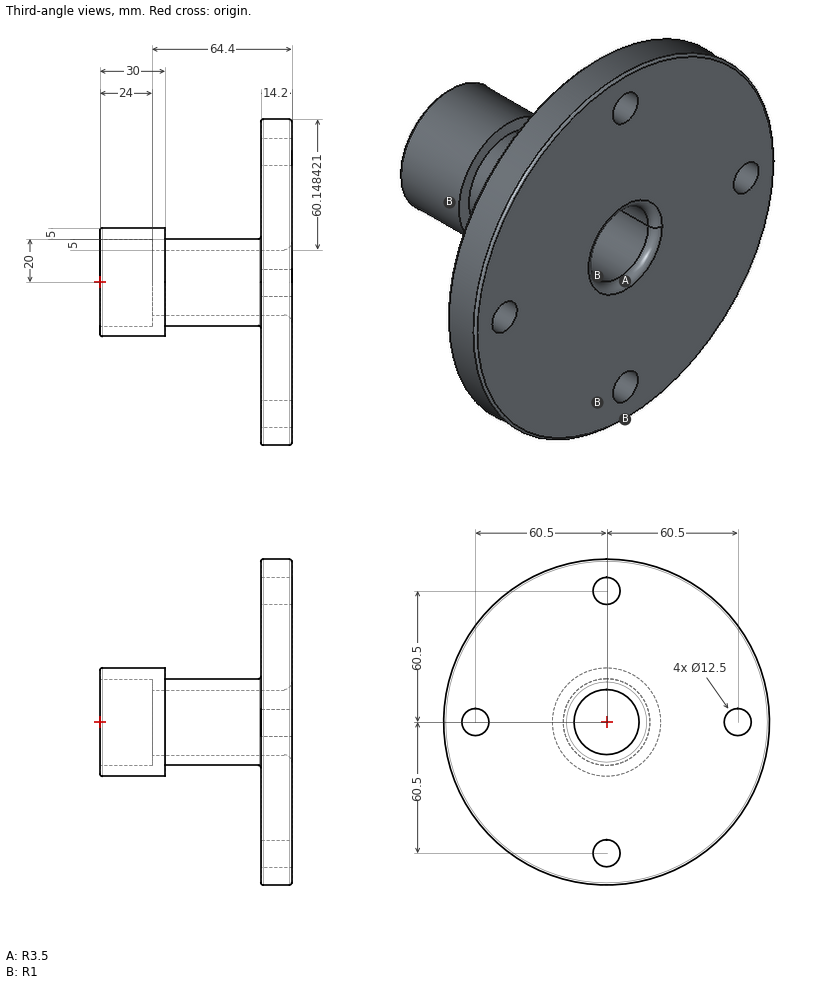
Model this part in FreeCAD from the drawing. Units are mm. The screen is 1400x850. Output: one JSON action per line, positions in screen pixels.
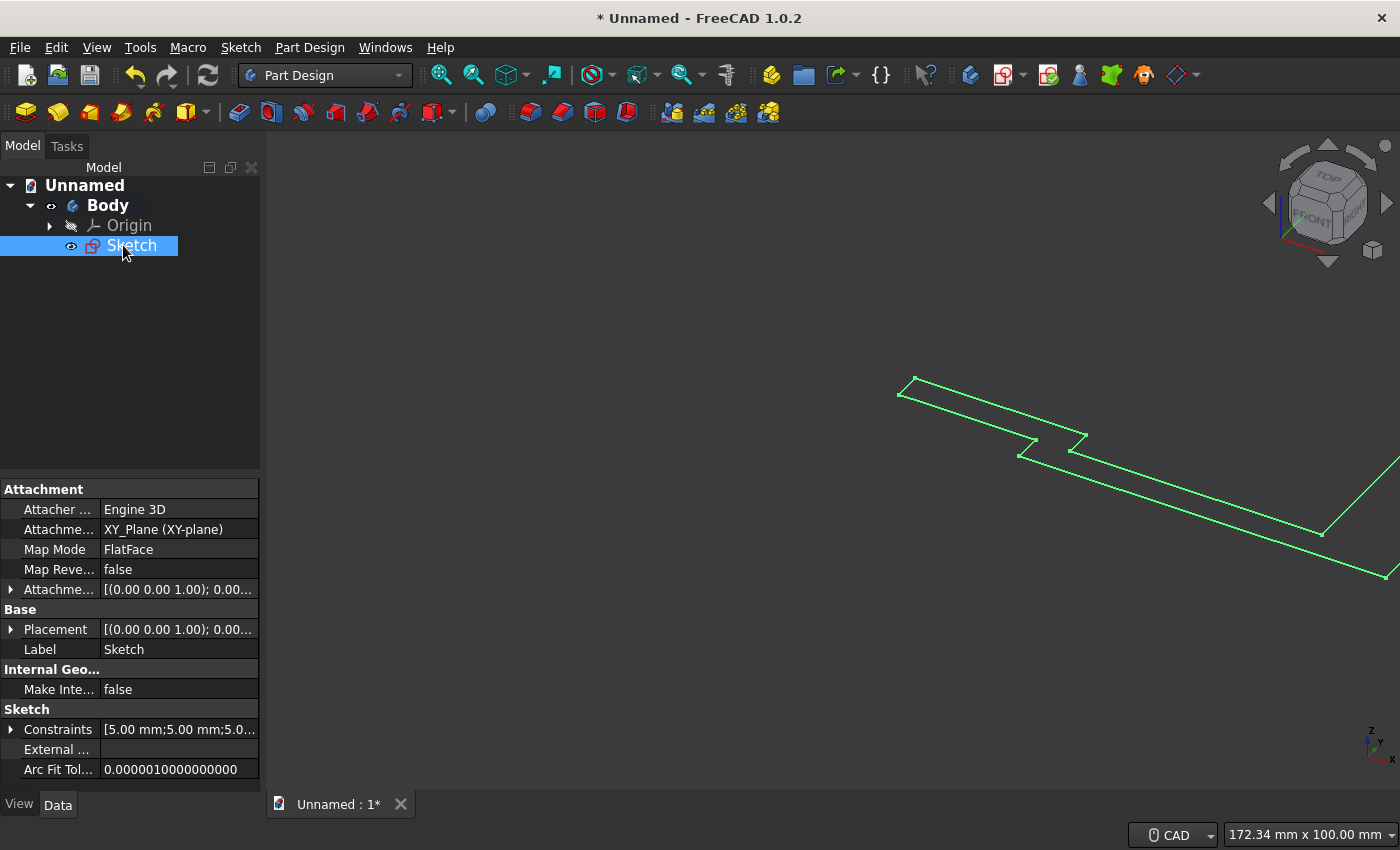
{"action": "left_click", "coordinate": [58, 112]}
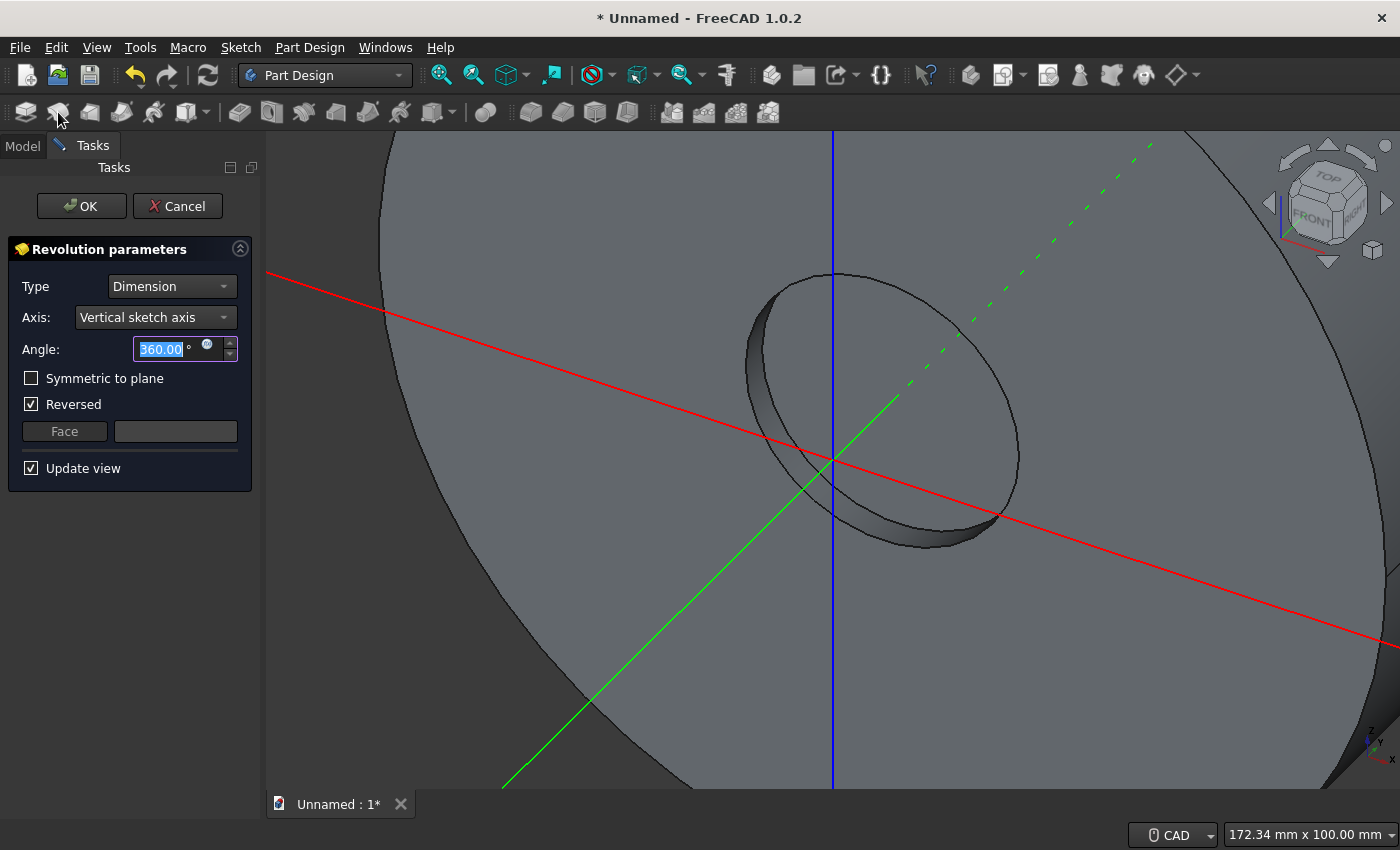
{"action": "left_click", "coordinate": [156, 318]}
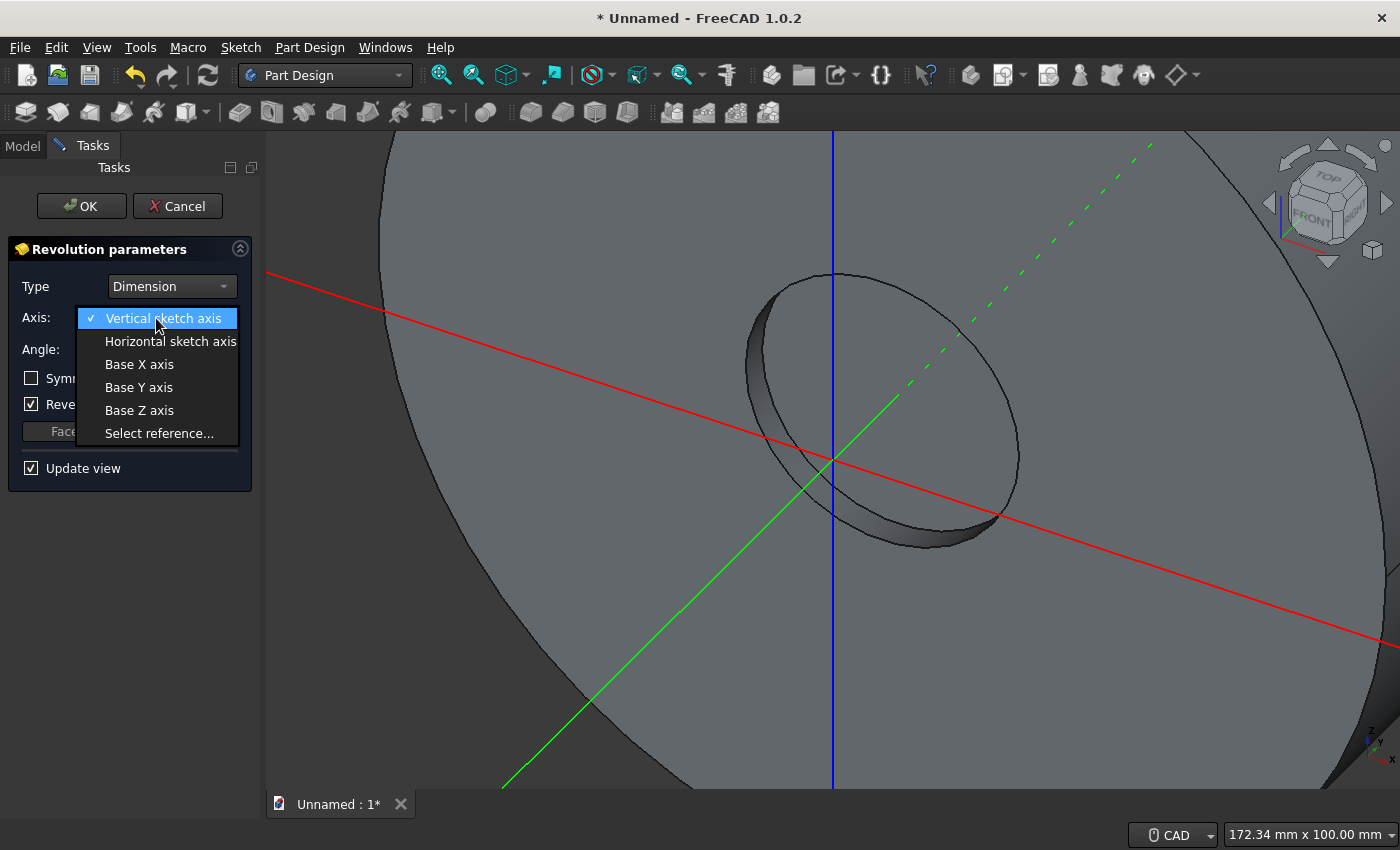
{"action": "left_click", "coordinate": [156, 342]}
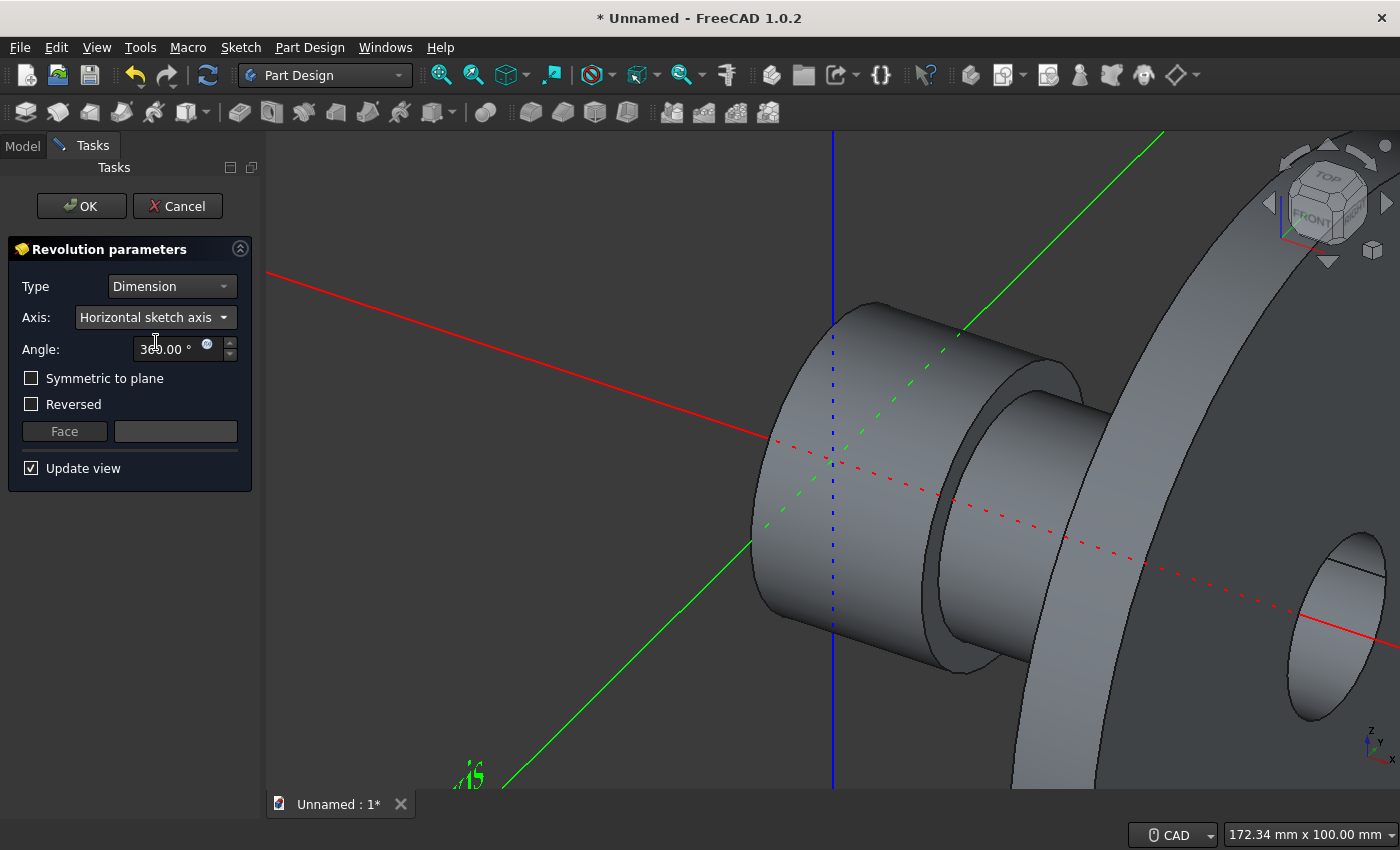
{"action": "left_click", "coordinate": [82, 206]}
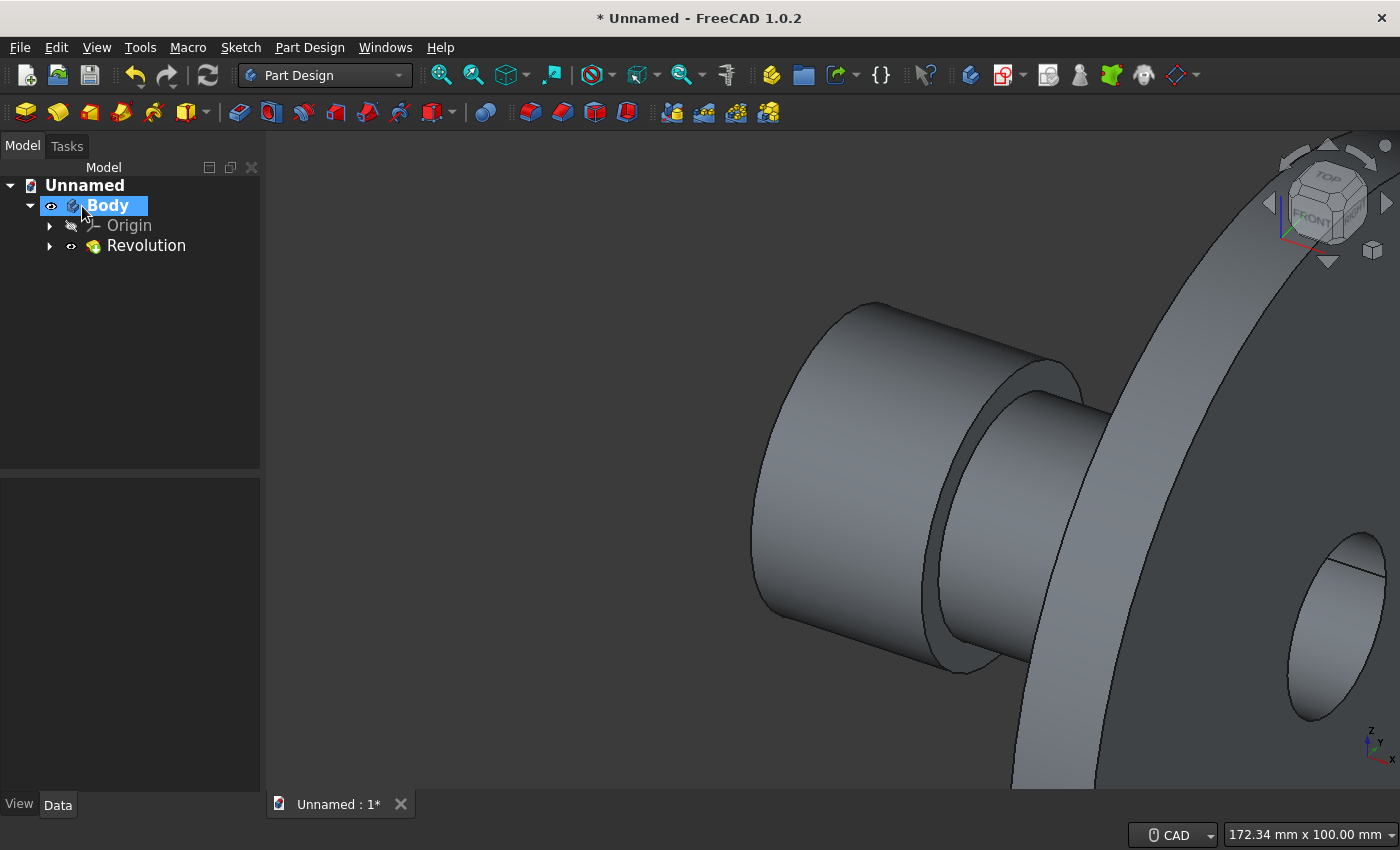
{"action": "key", "text": "v f"}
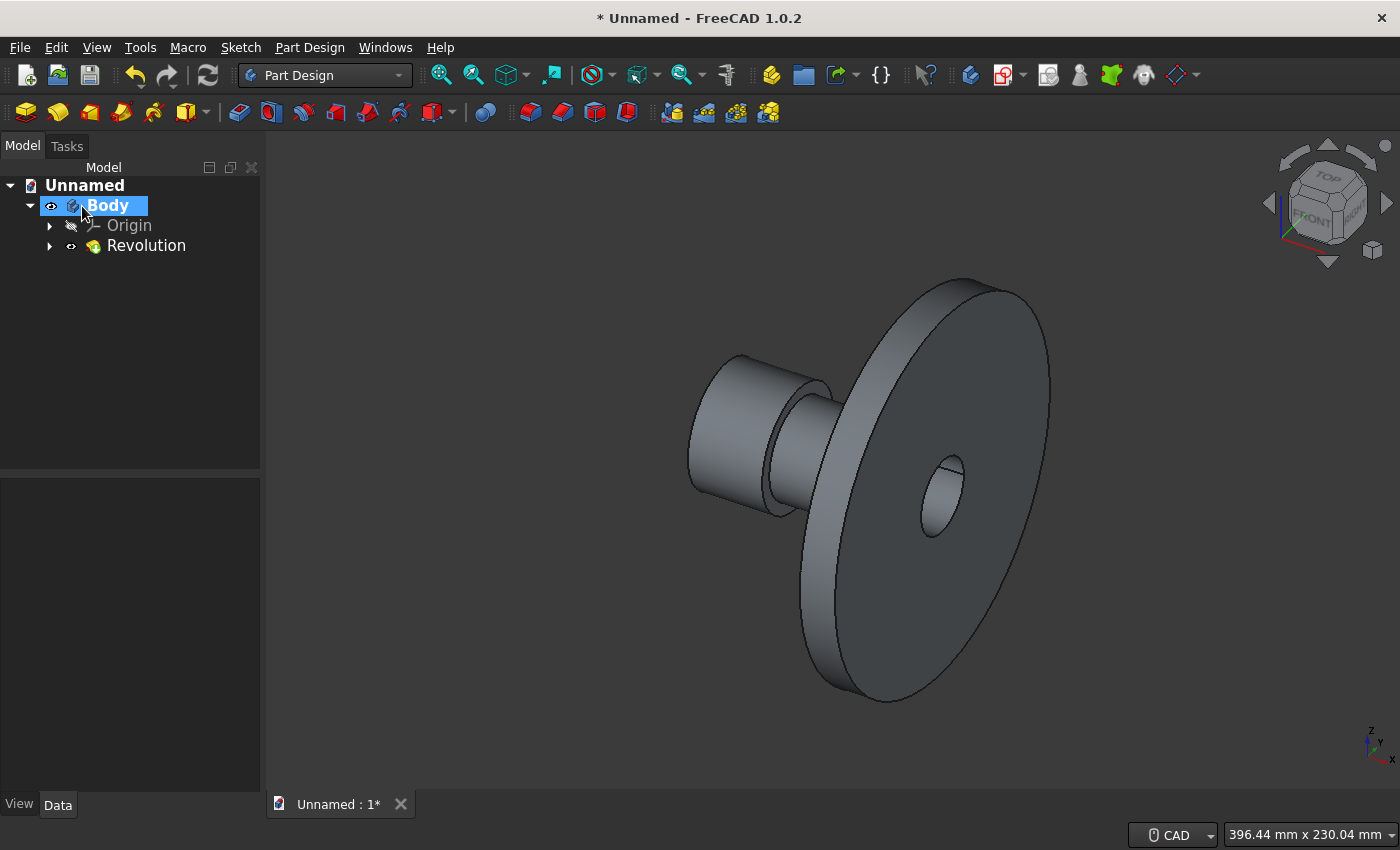
{"action": "key", "text": "6"}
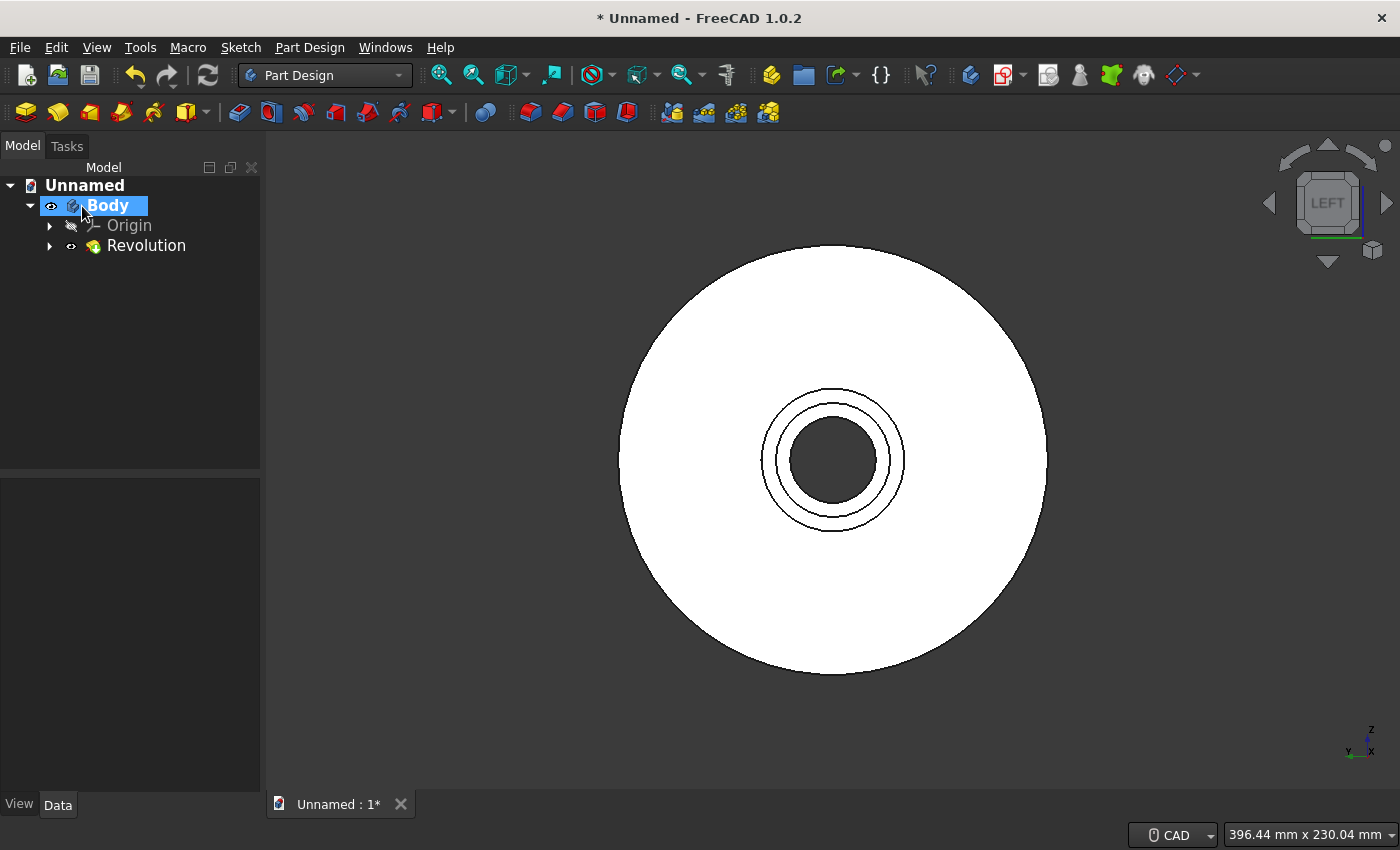
{"action": "left_click", "coordinate": [710, 398]}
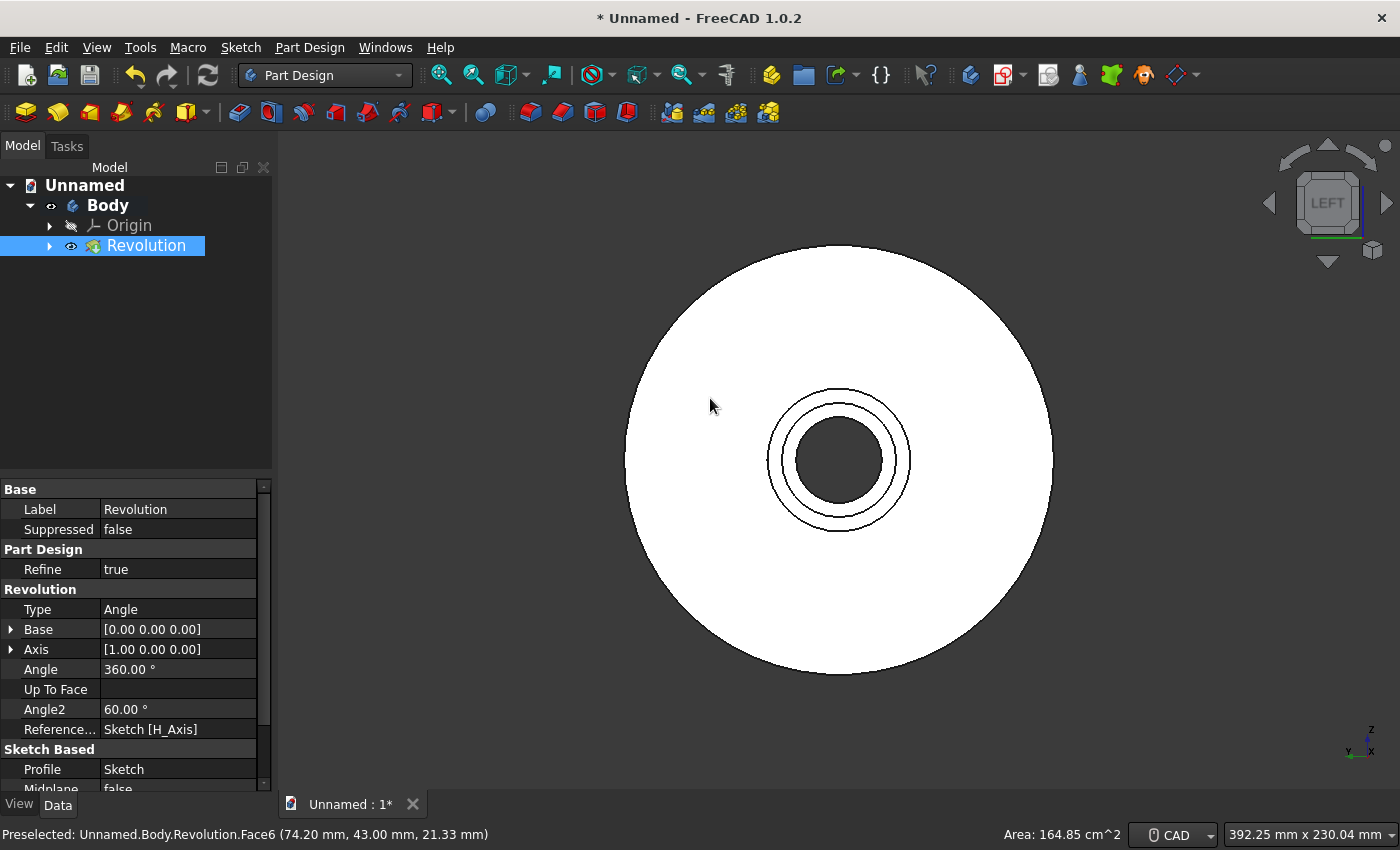
{"action": "left_click", "coordinate": [1004, 76]}